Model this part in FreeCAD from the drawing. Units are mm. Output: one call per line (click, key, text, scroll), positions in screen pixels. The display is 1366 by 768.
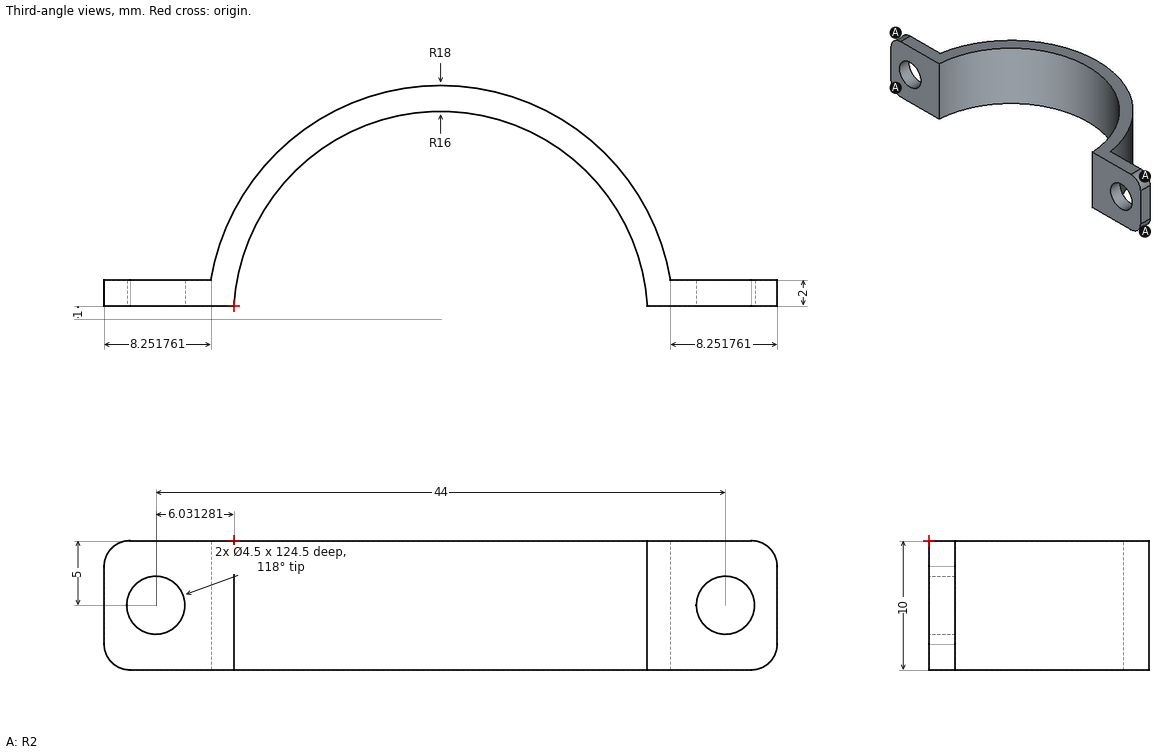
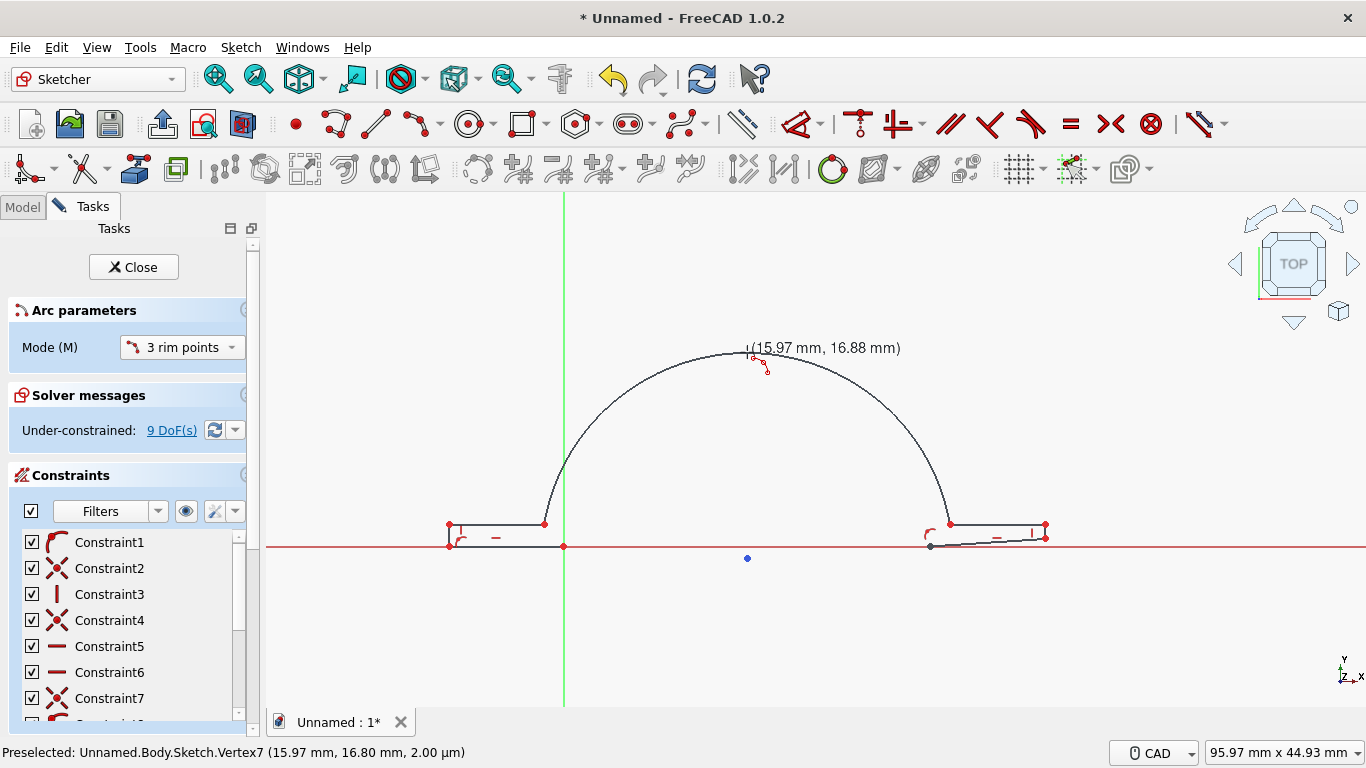
click(564, 547)
click(930, 547)
click(747, 375)
key(Escape)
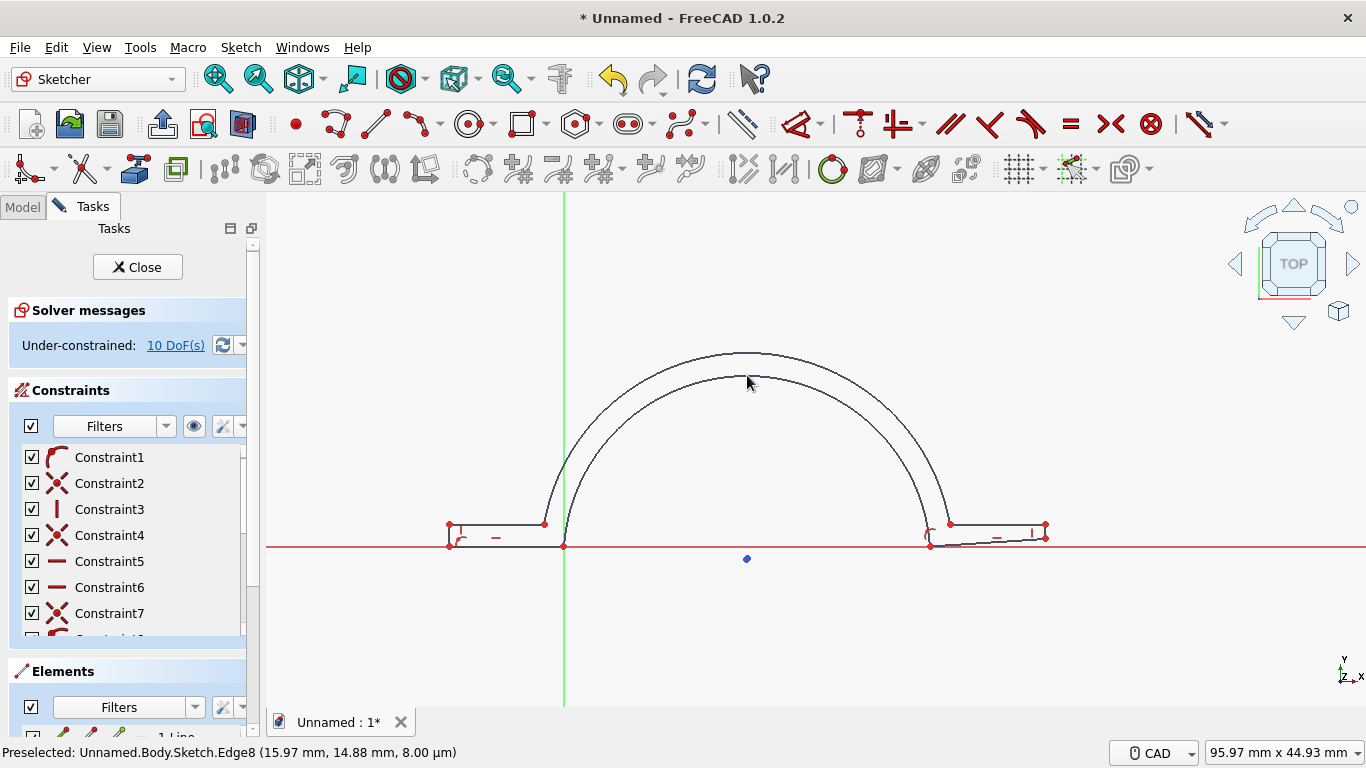
click(965, 544)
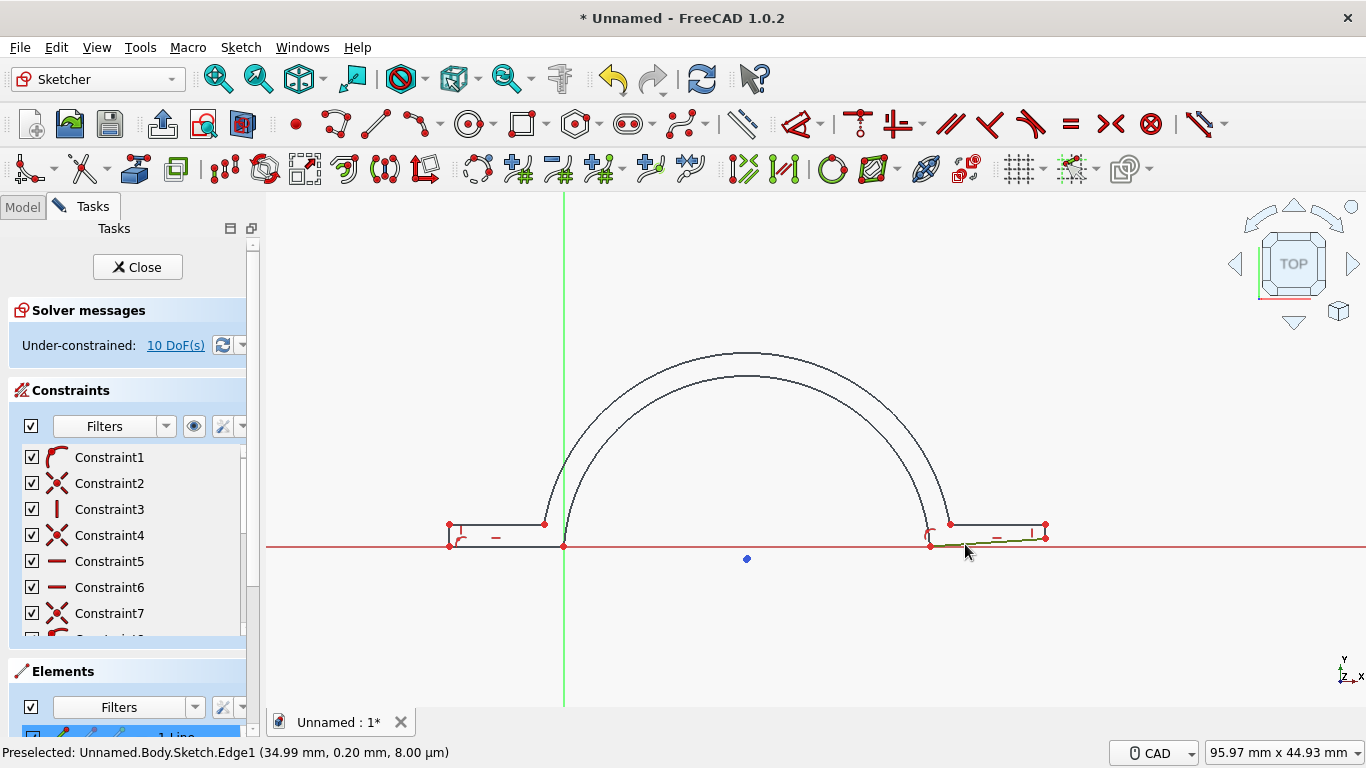
click(924, 124)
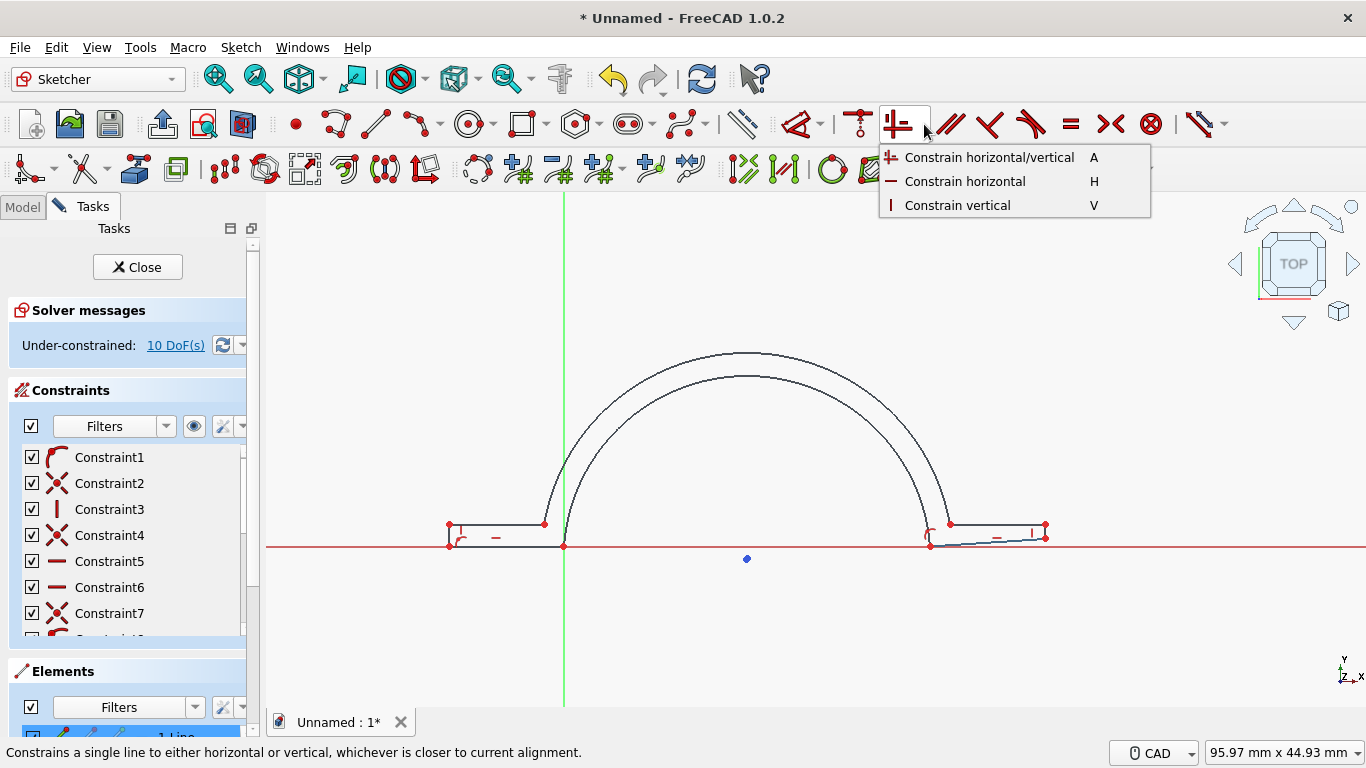
click(1015, 181)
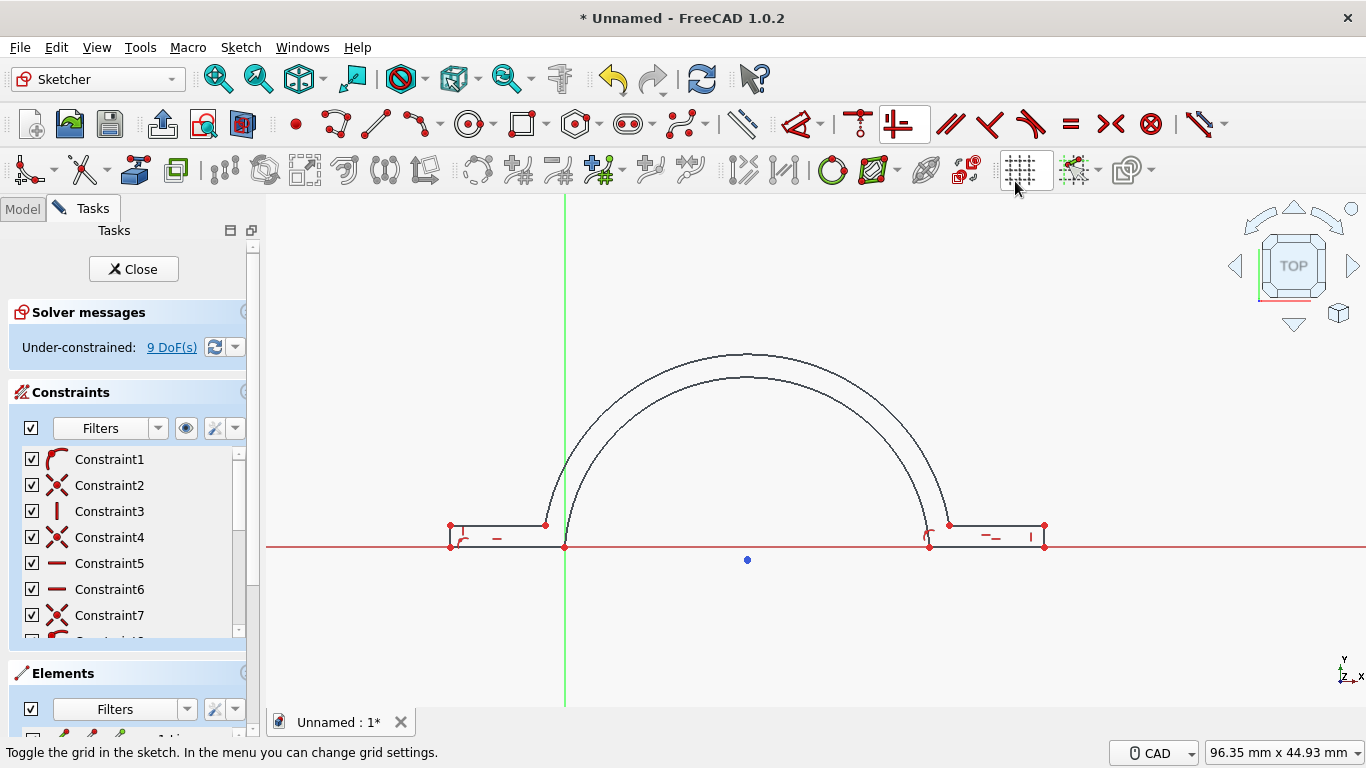
click(857, 386)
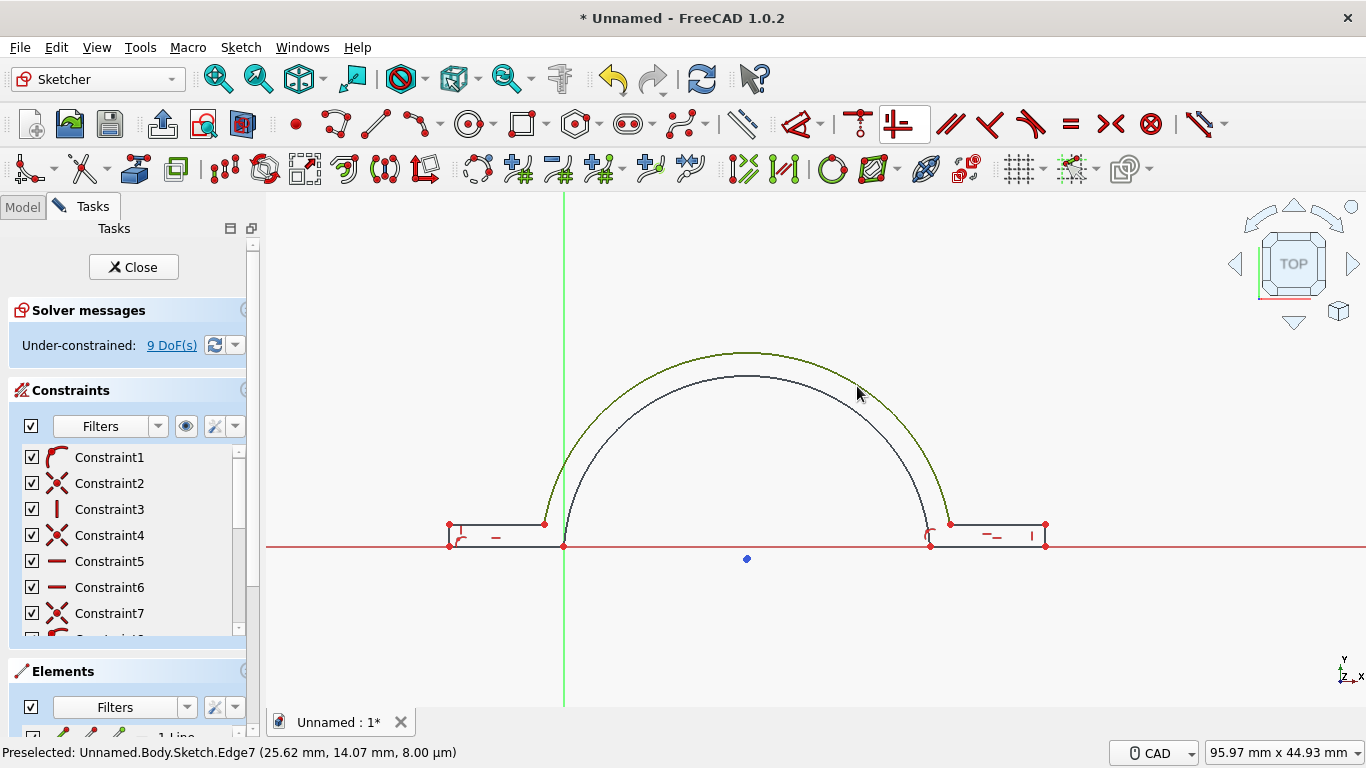
click(851, 408)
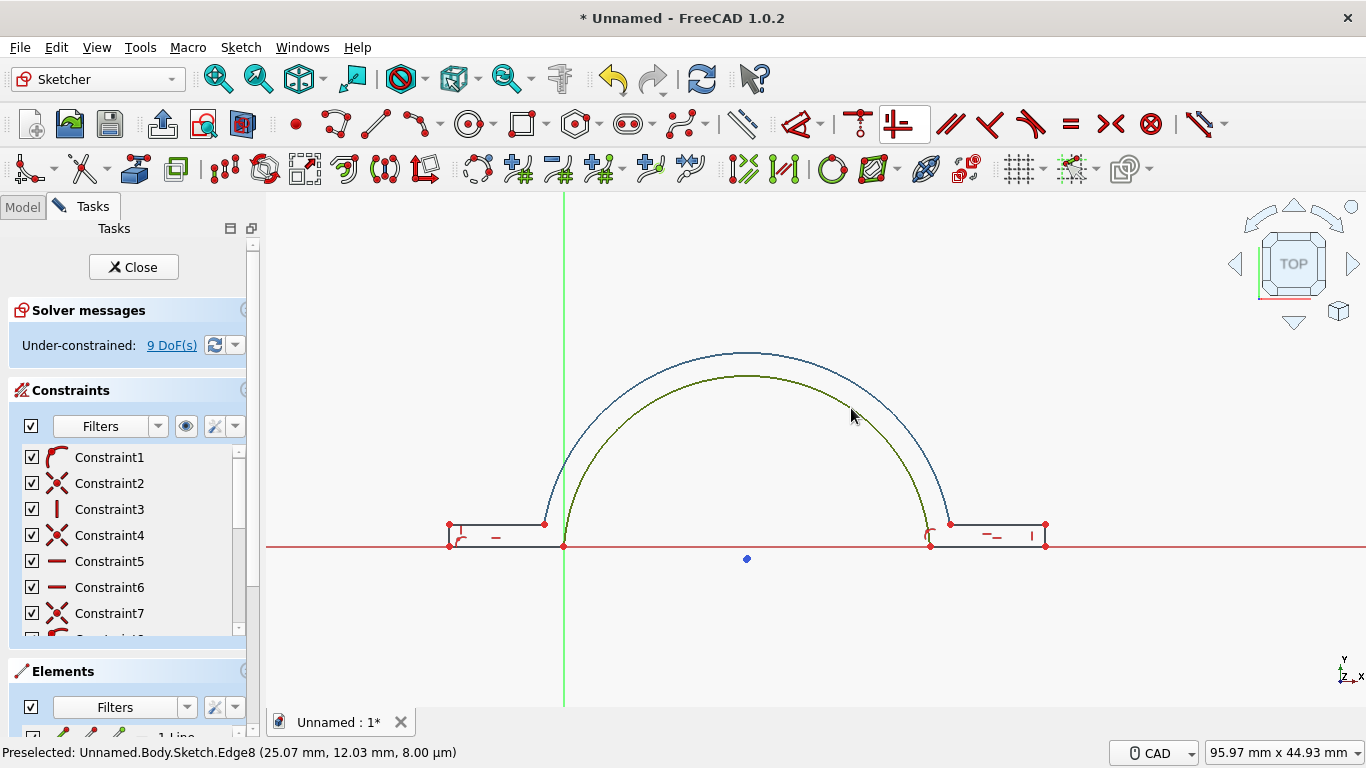
click(858, 124)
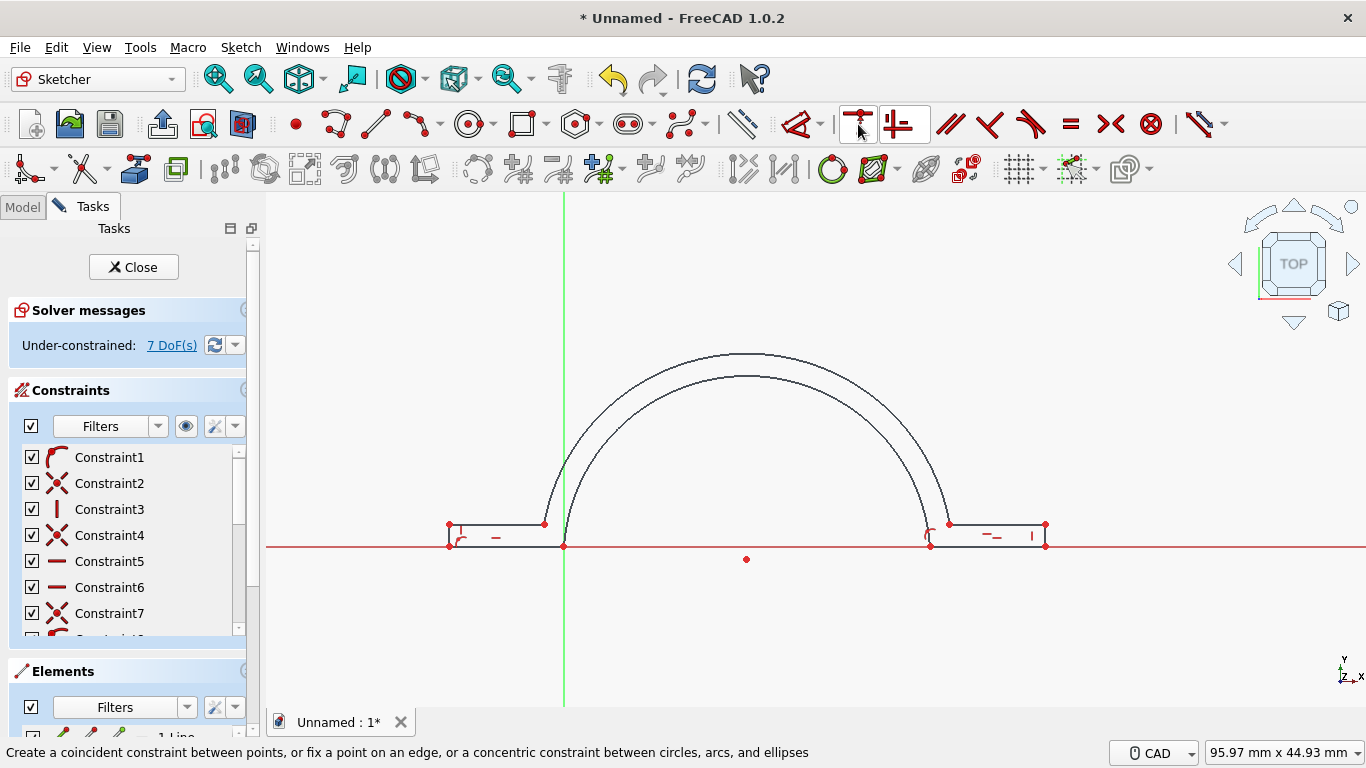
click(856, 385)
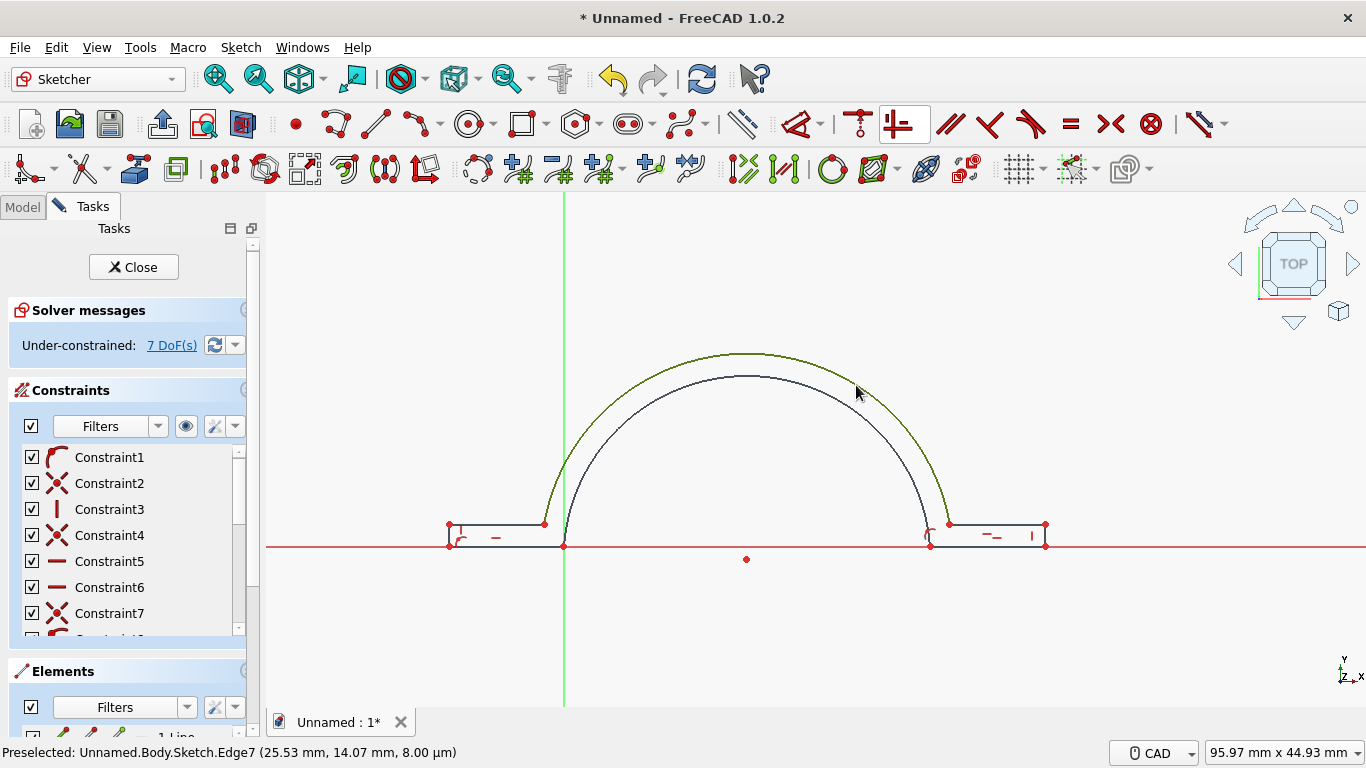
key(k)
key(r)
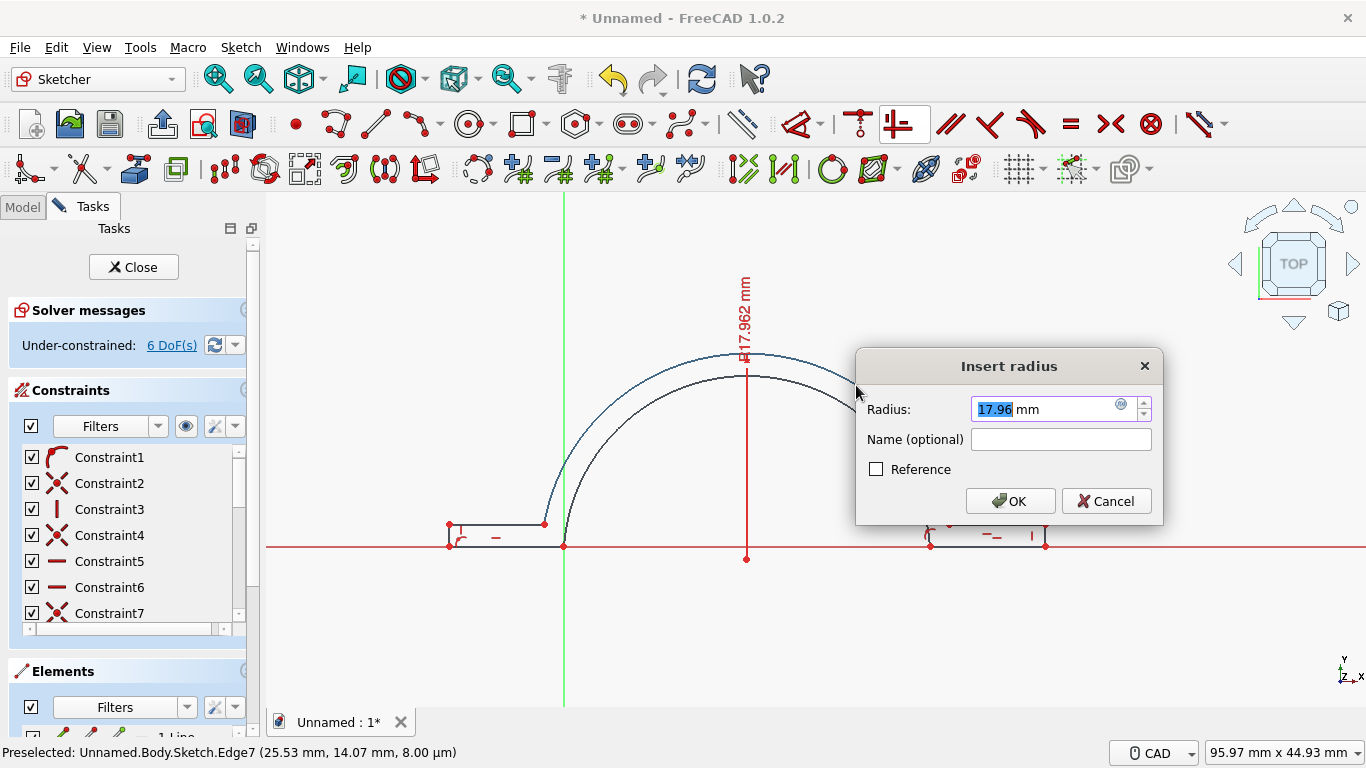
text(18)
key(Return)